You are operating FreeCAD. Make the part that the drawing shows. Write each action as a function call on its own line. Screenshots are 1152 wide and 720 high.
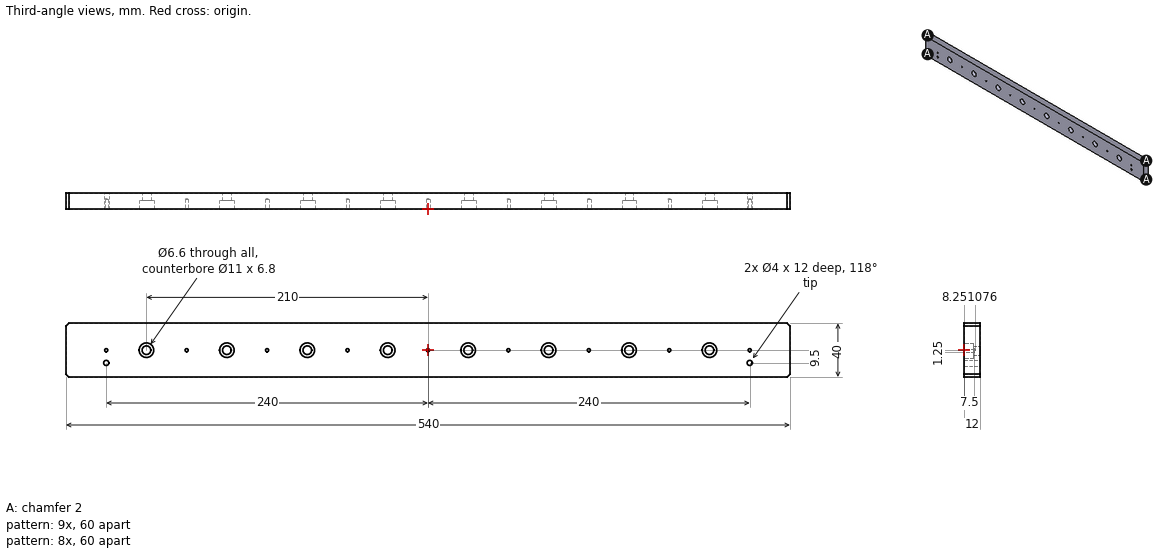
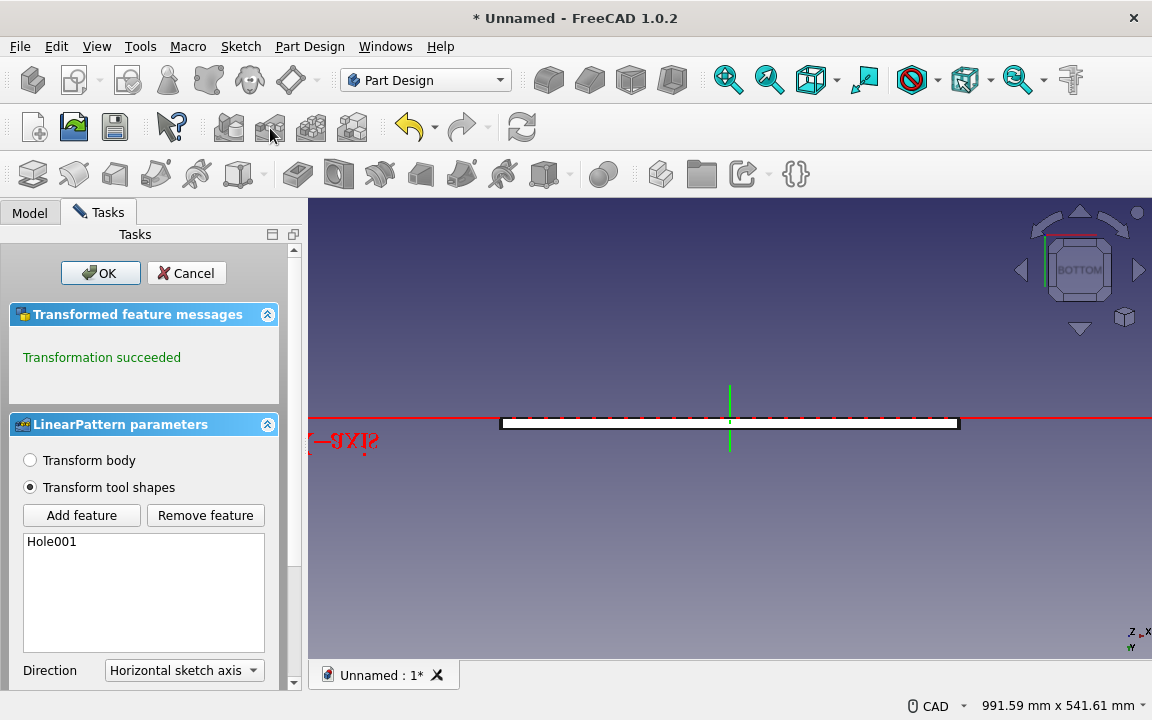
click(185, 670)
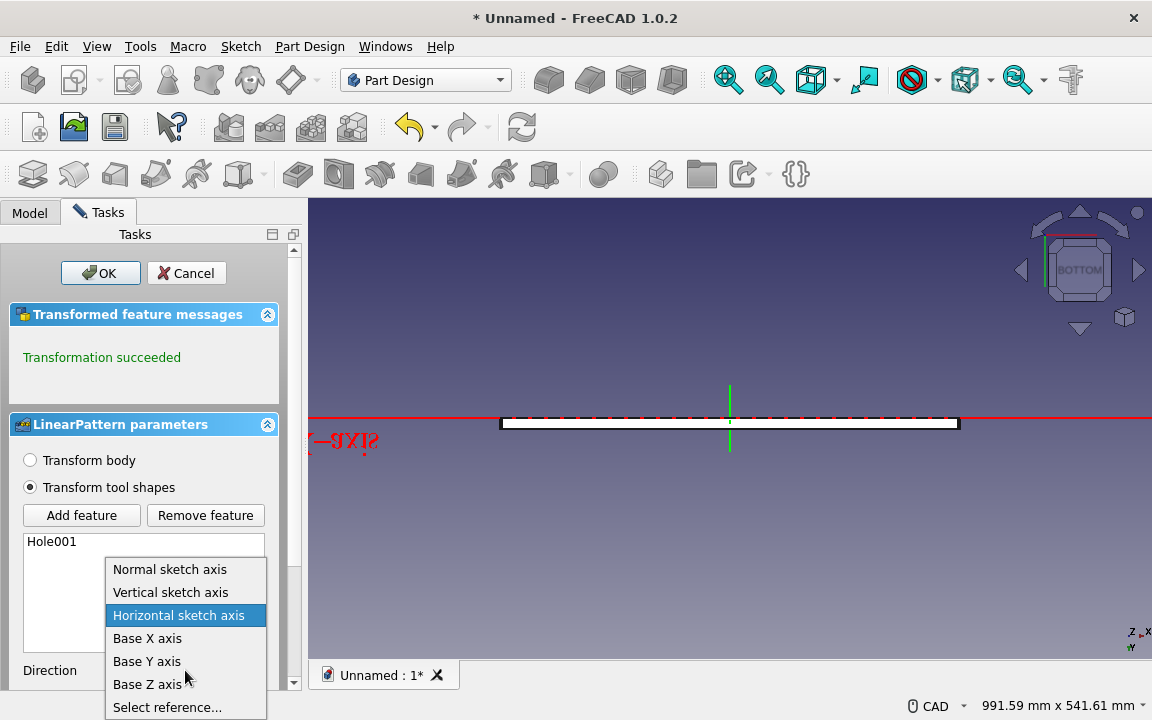
click(184, 638)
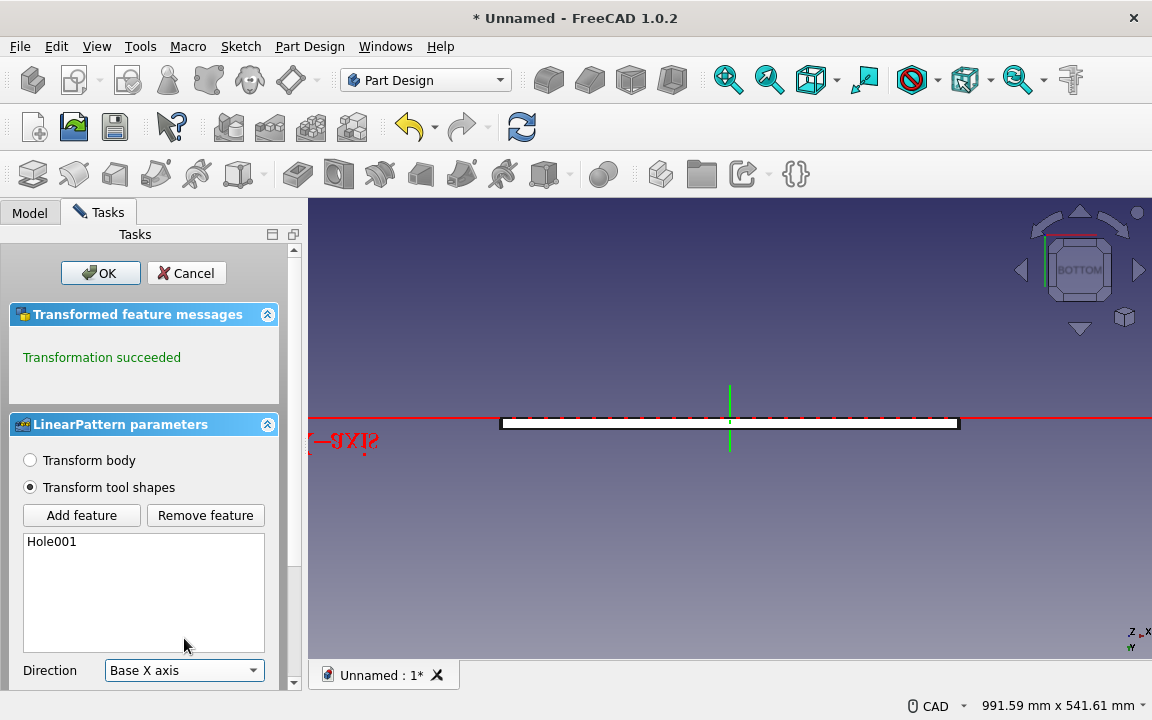
scroll(294, 467, down, 2)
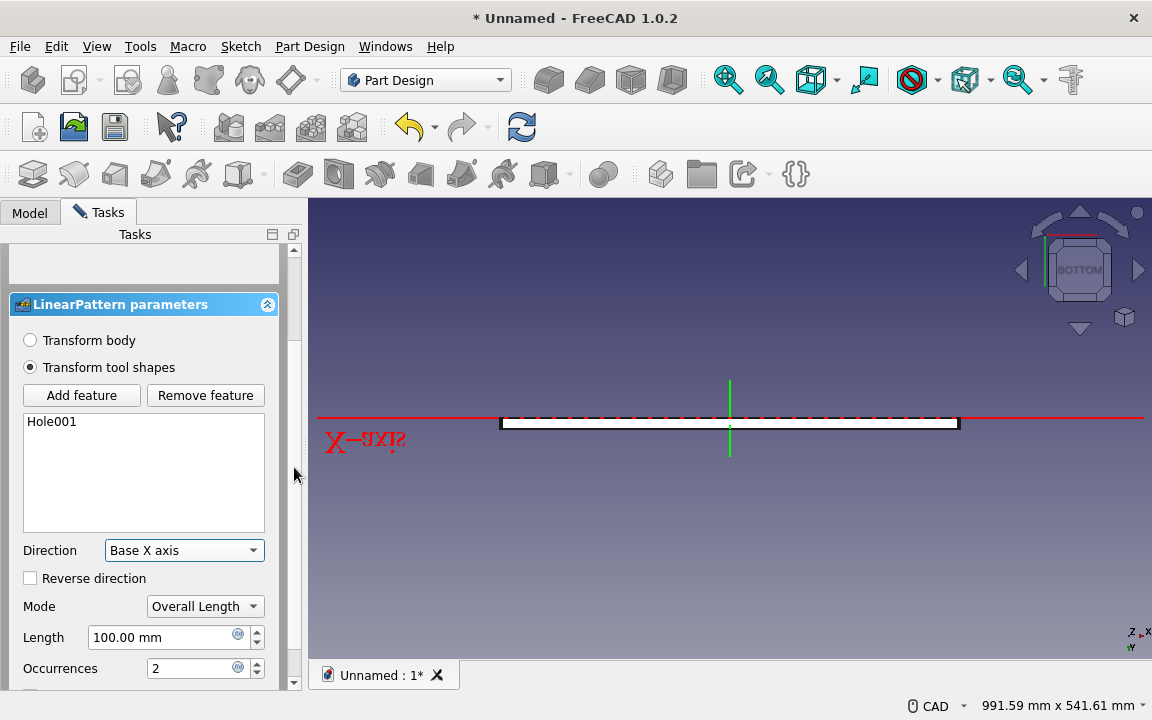
click(206, 606)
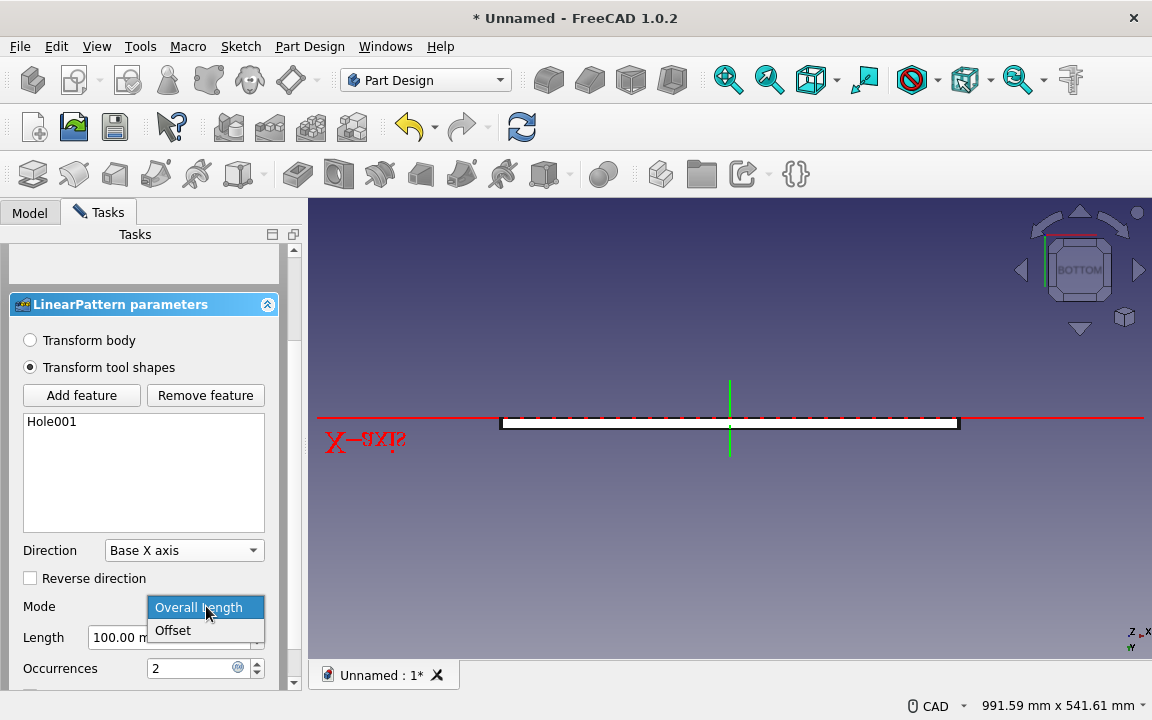
click(204, 630)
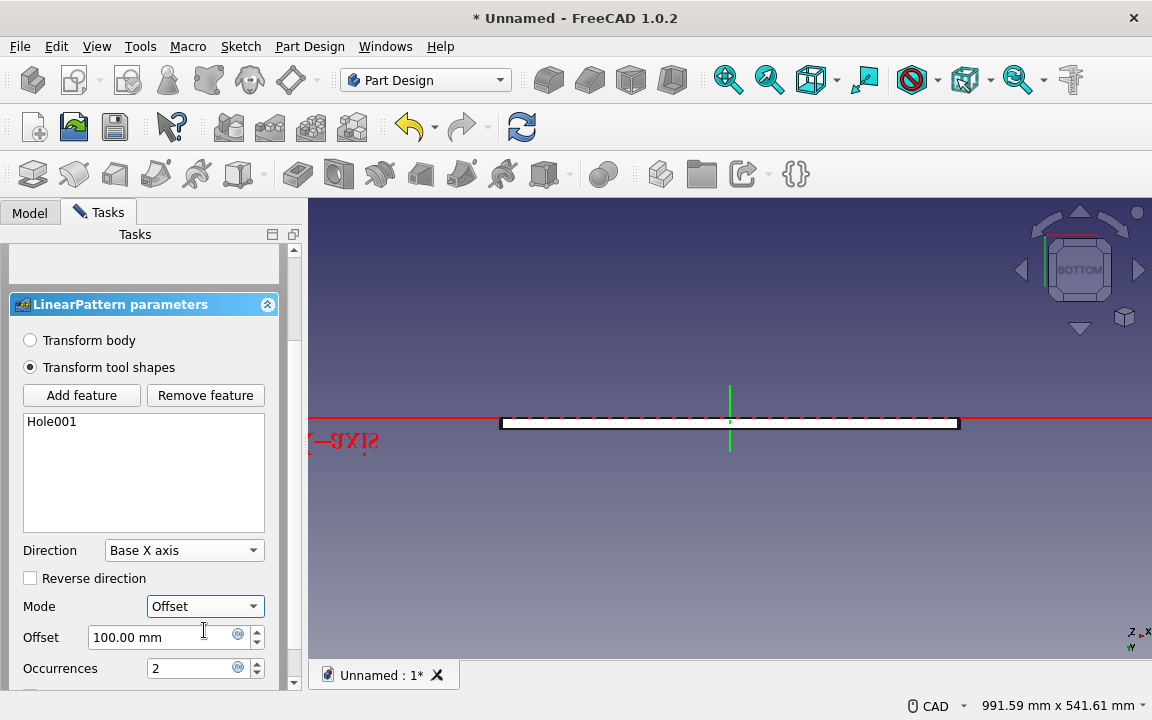
triple_click(170, 638)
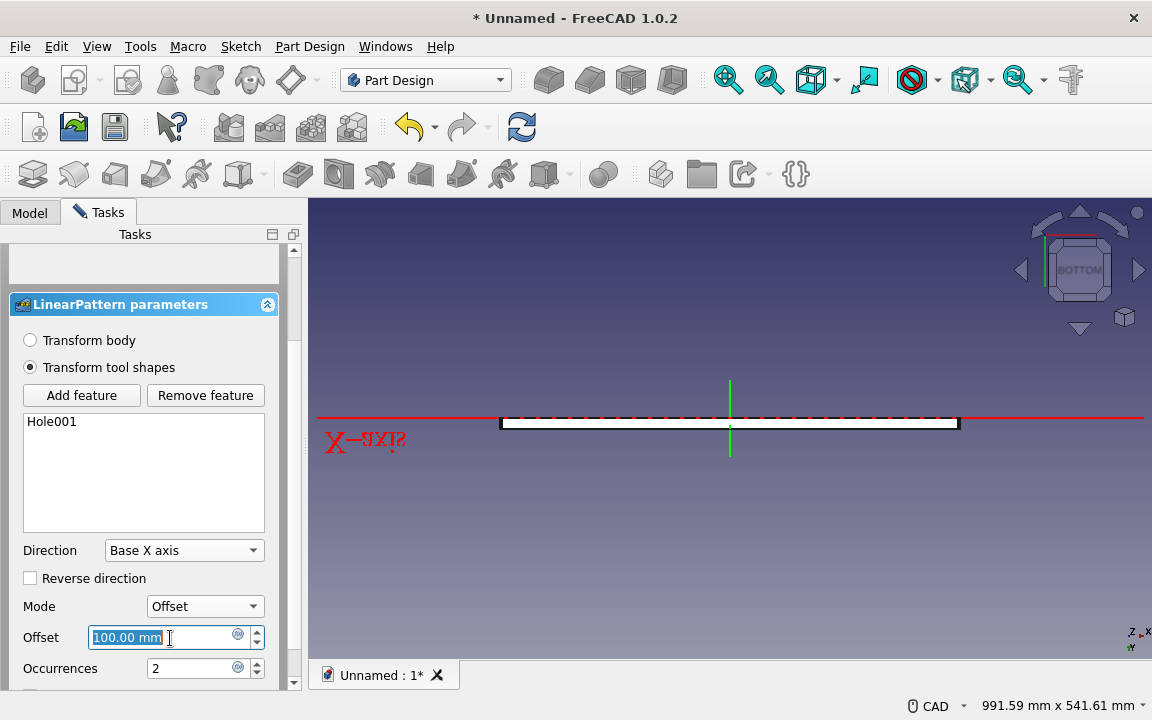
text(60)
key(Tab)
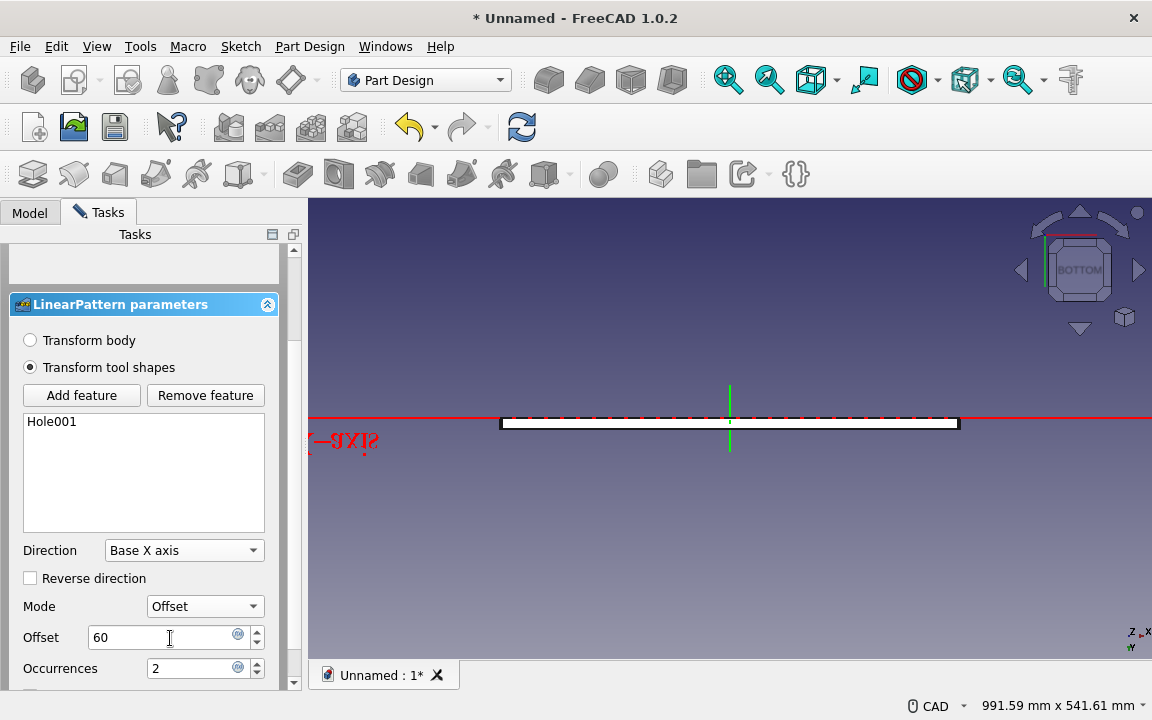
triple_click(199, 668)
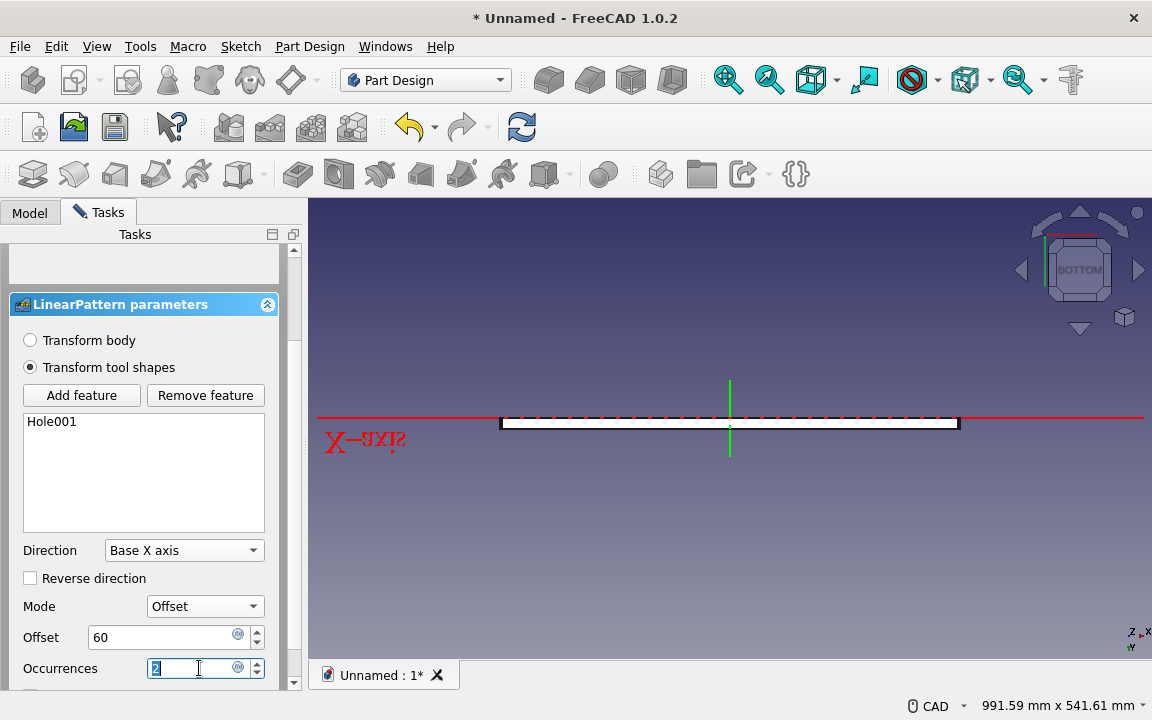
text(8)
key(Tab)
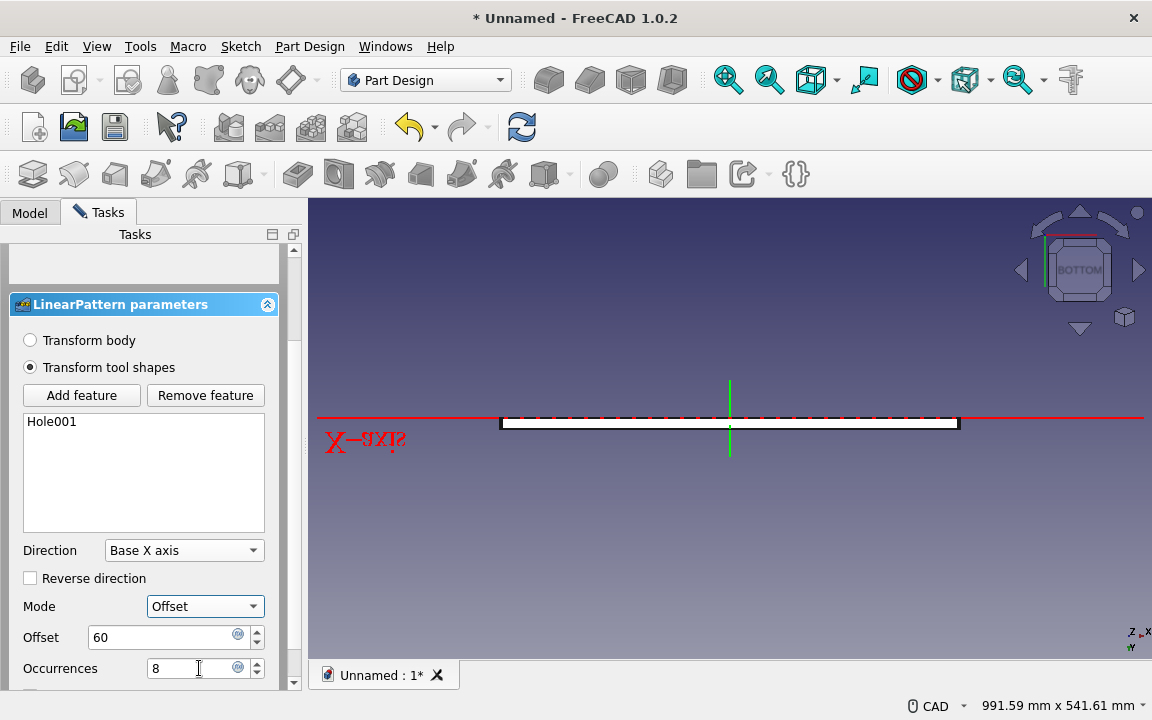
scroll(294, 467, up, 3)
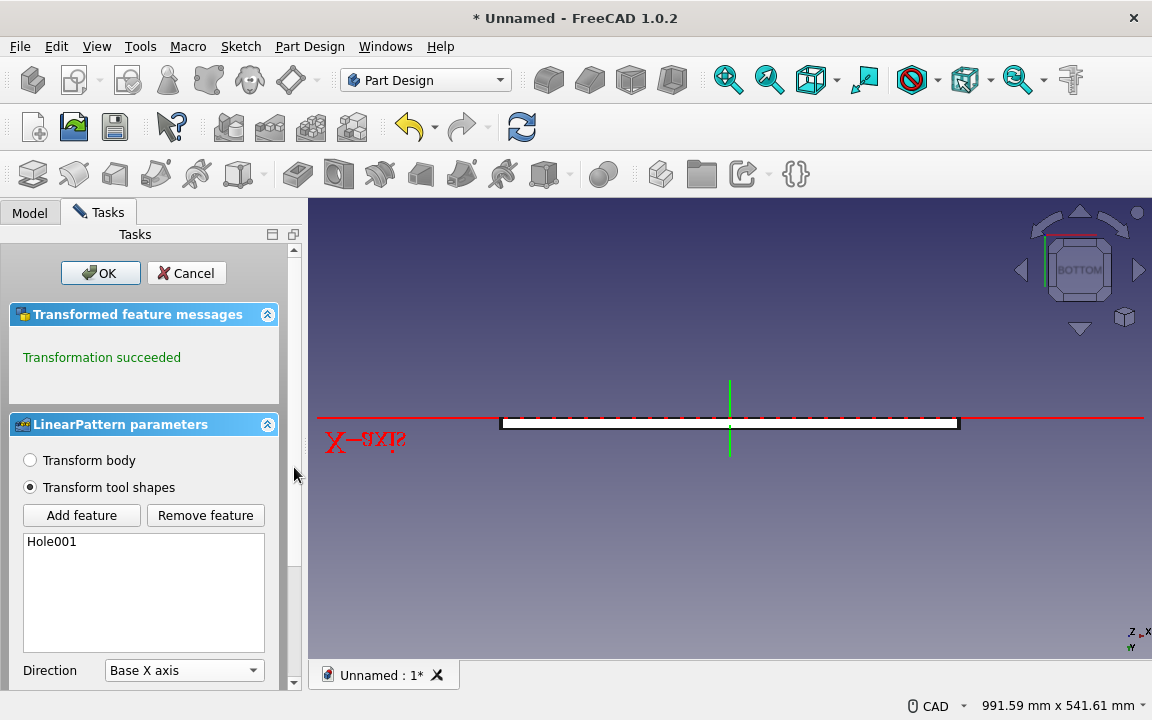
click(101, 273)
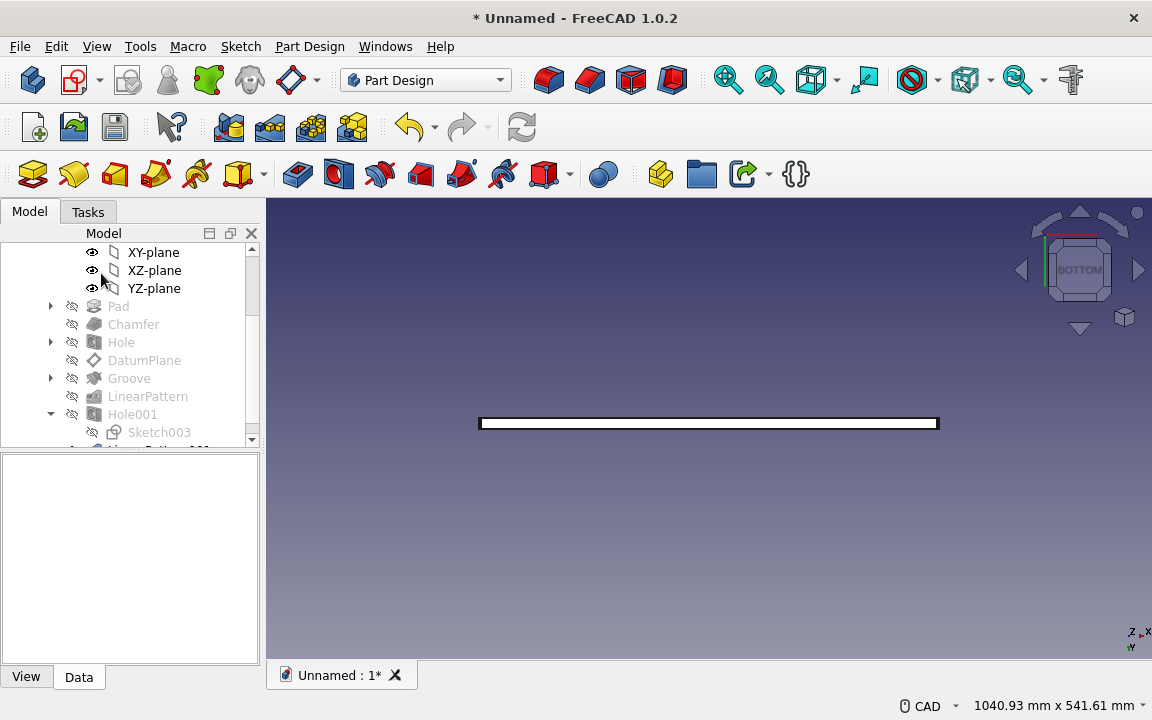
key(0)